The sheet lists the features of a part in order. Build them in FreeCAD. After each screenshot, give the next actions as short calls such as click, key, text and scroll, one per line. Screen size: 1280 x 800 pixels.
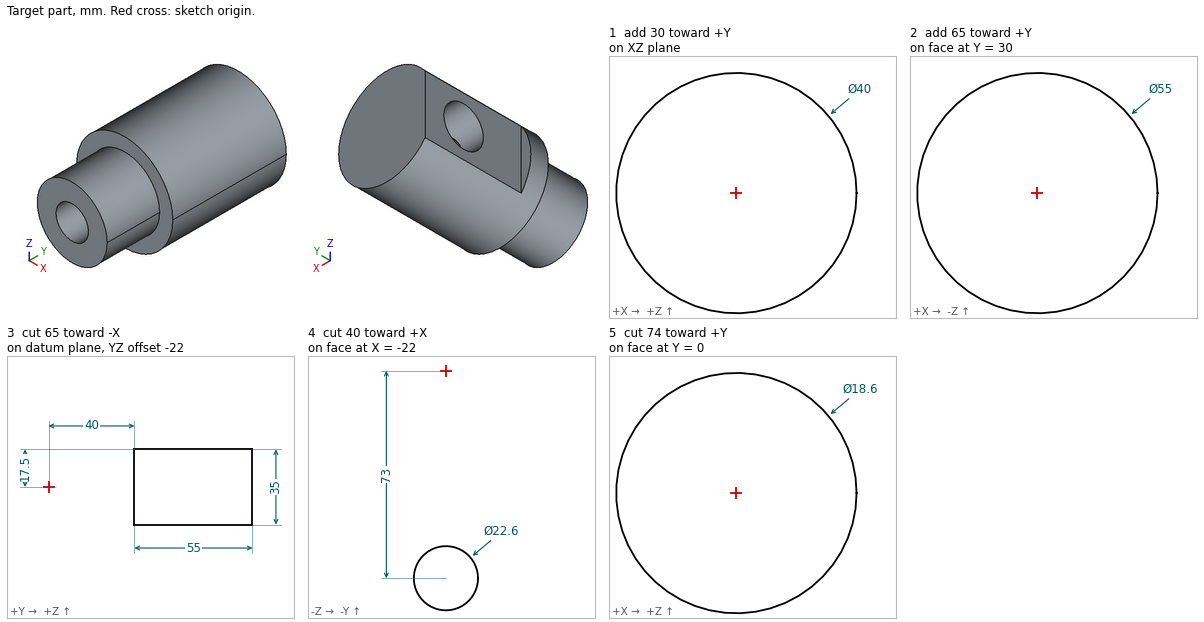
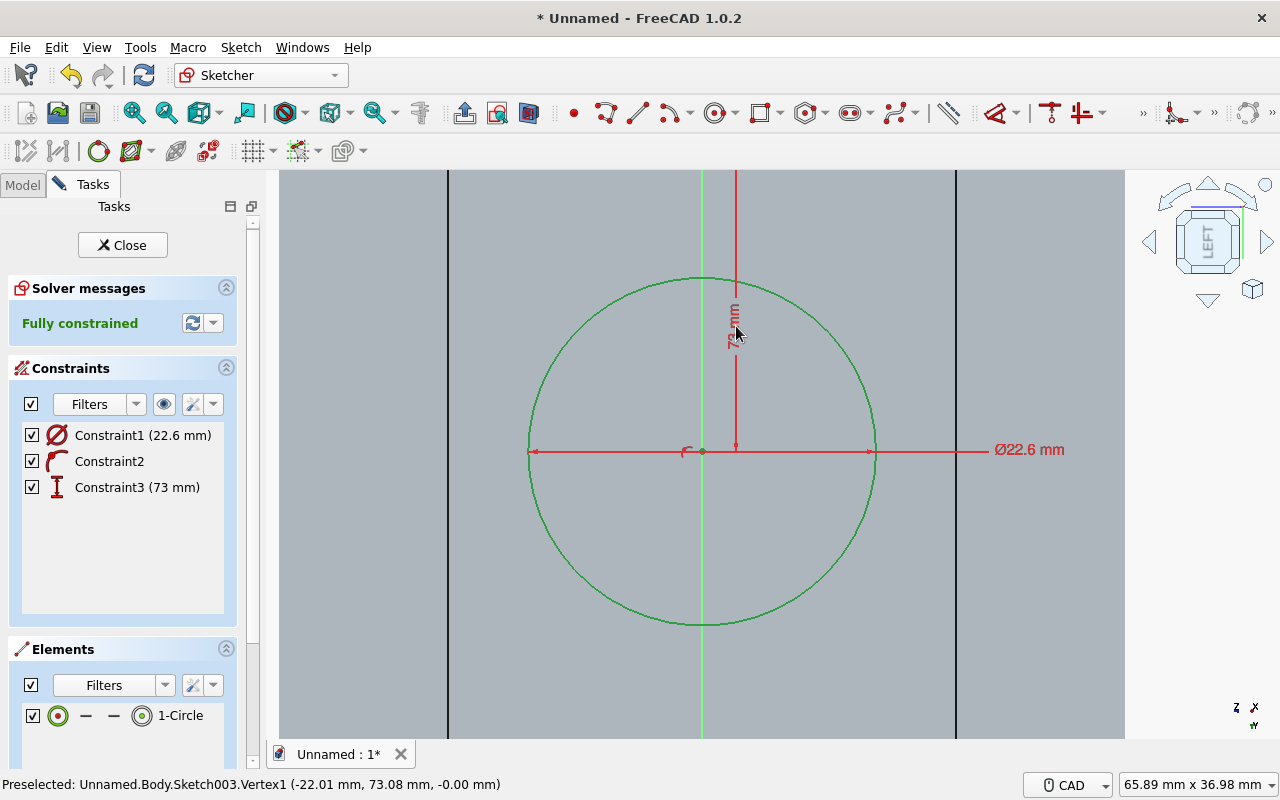
click(123, 245)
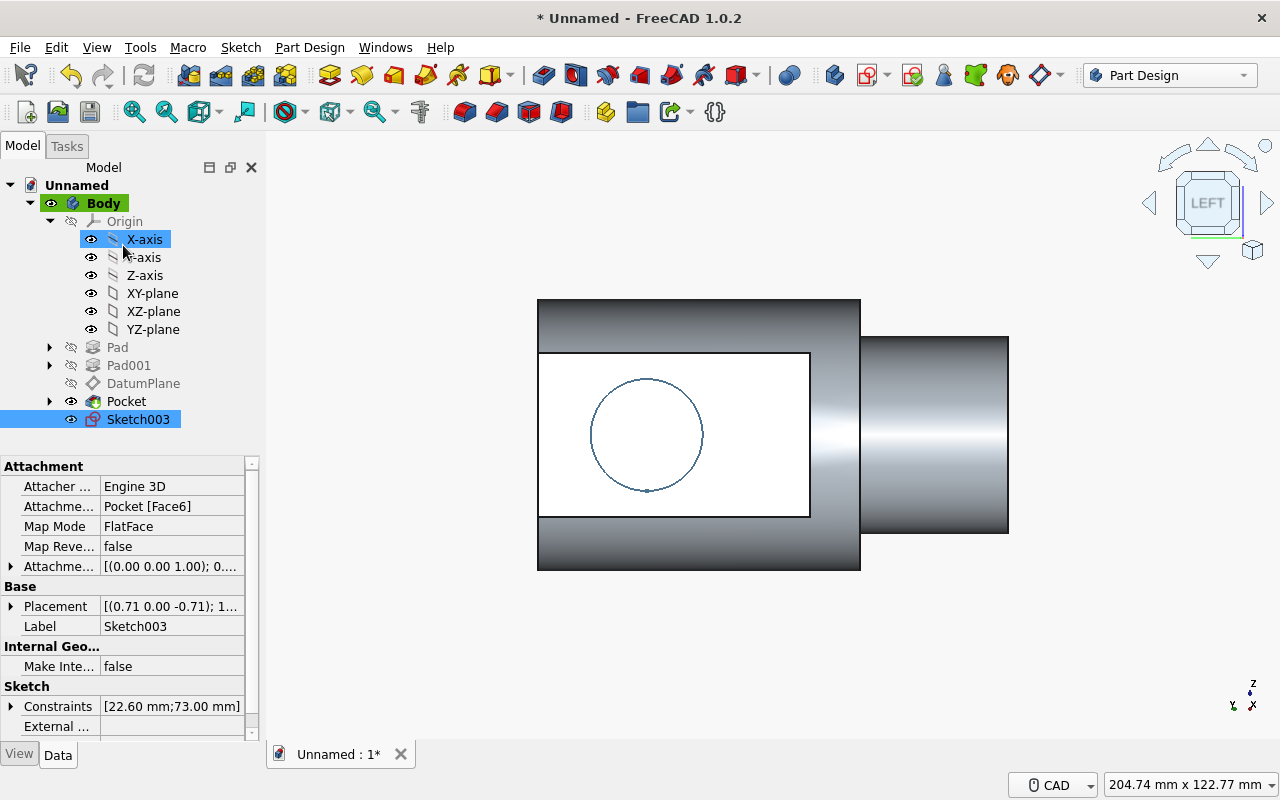
click(544, 76)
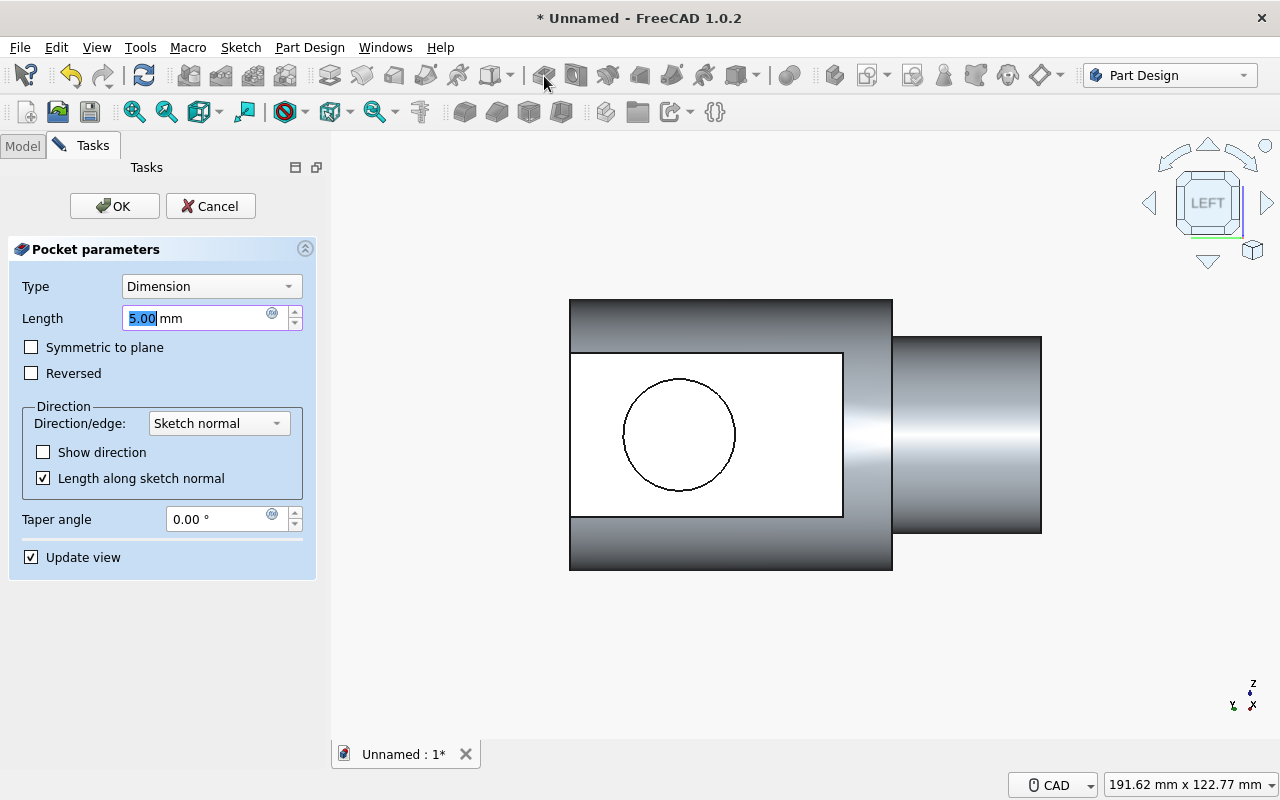
text(40)
key(Tab)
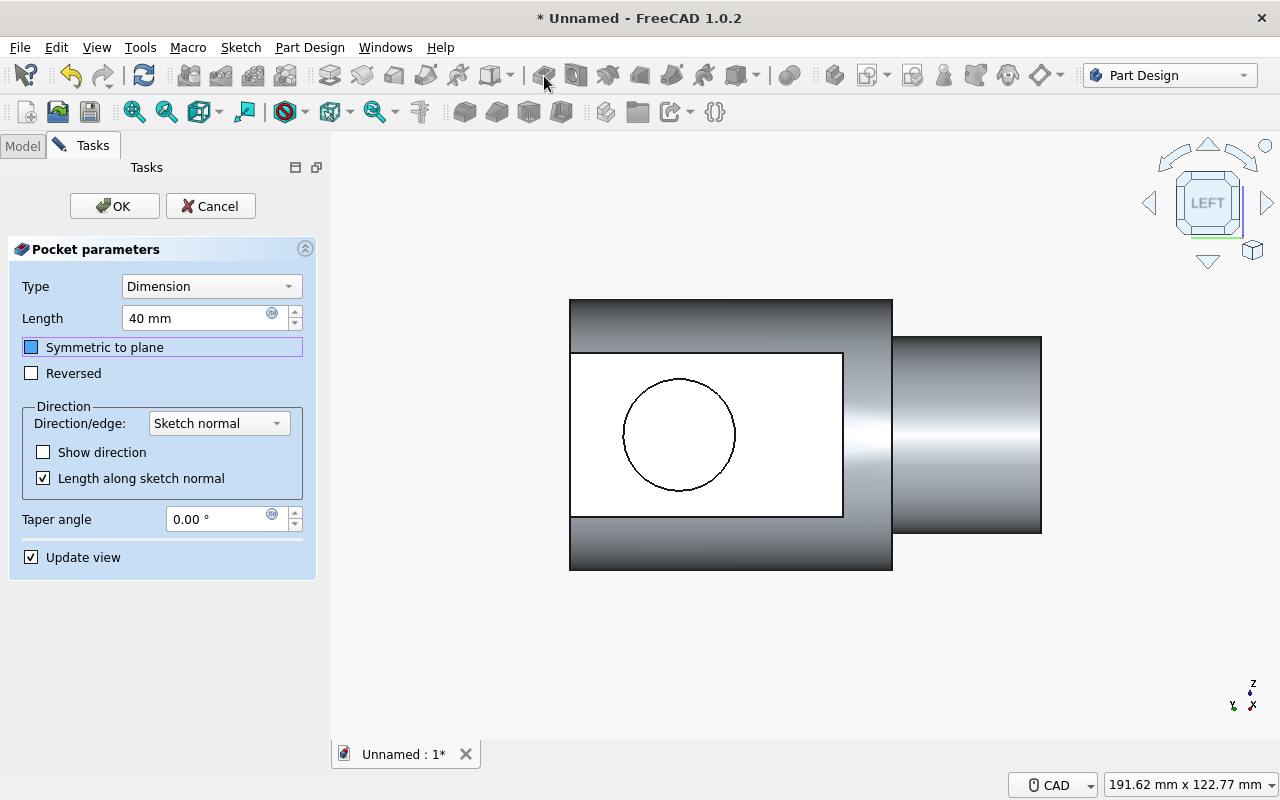
click(115, 206)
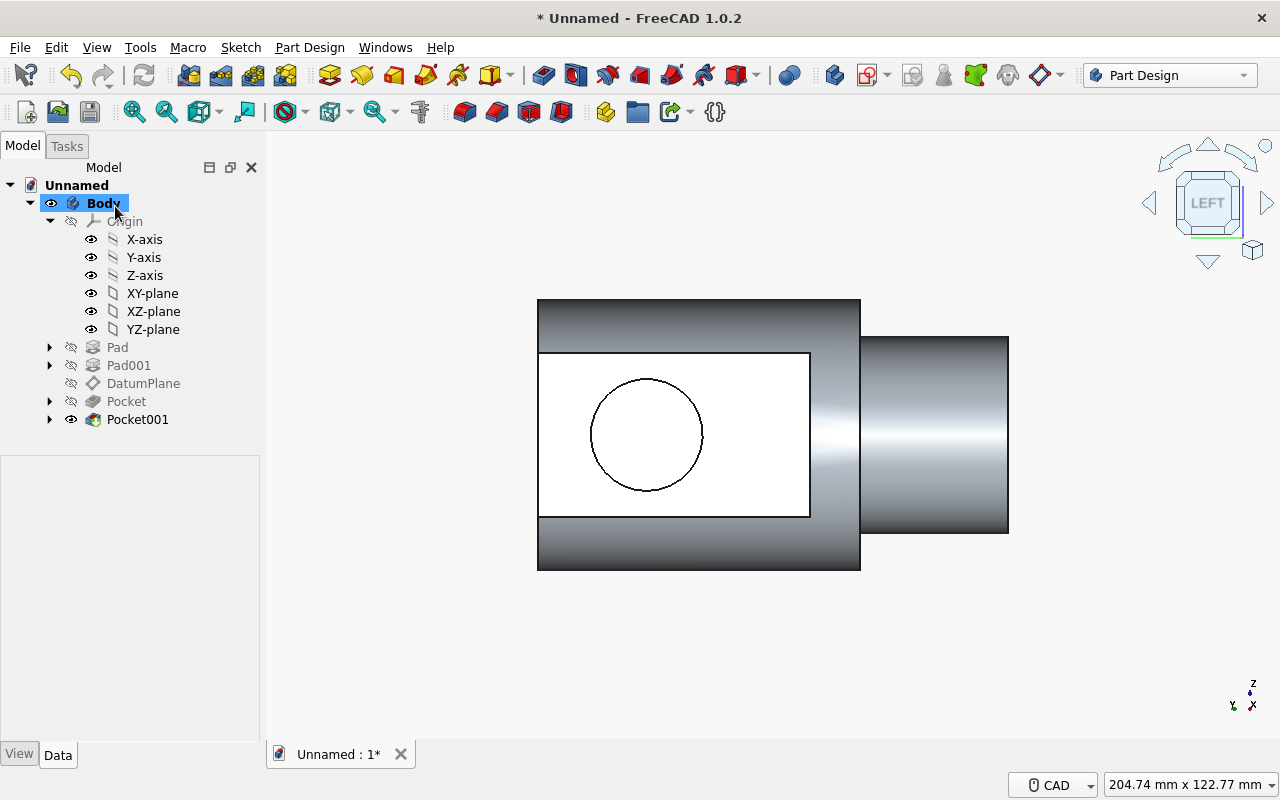
key(0)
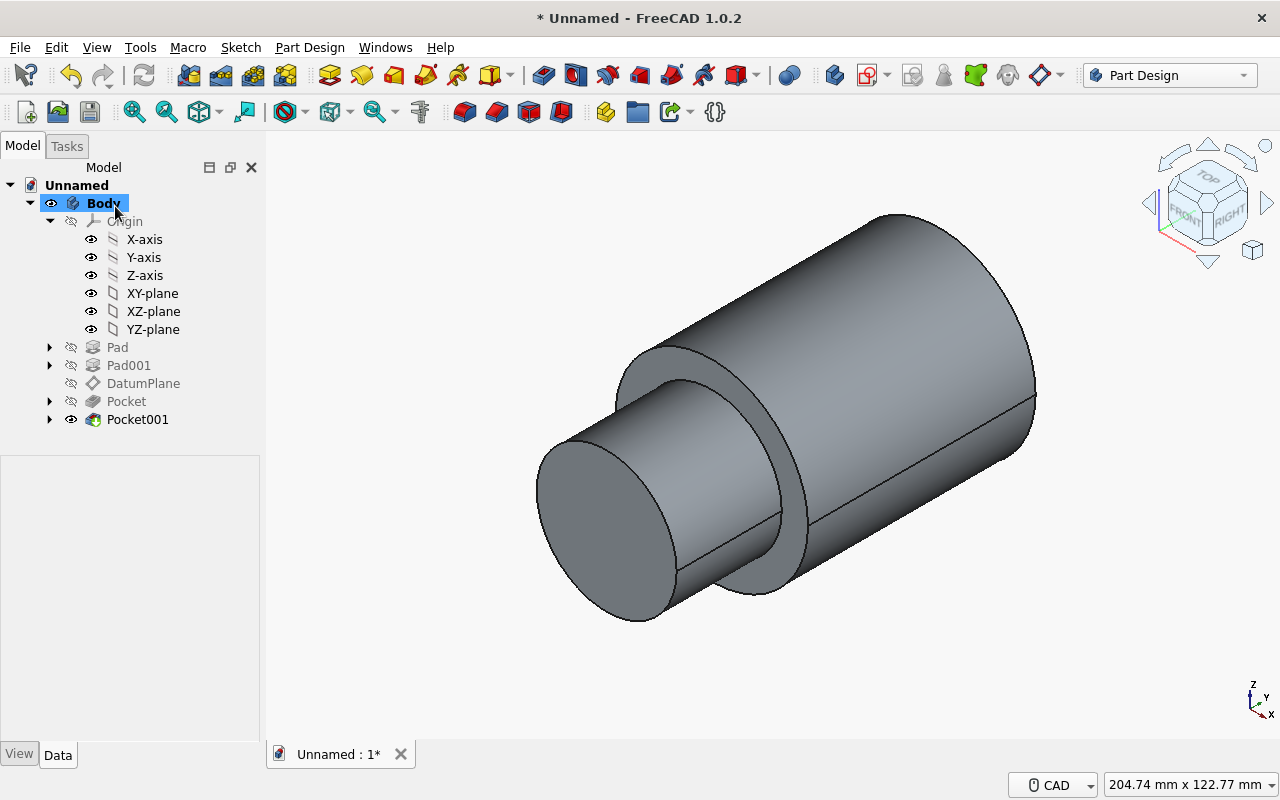
click(607, 530)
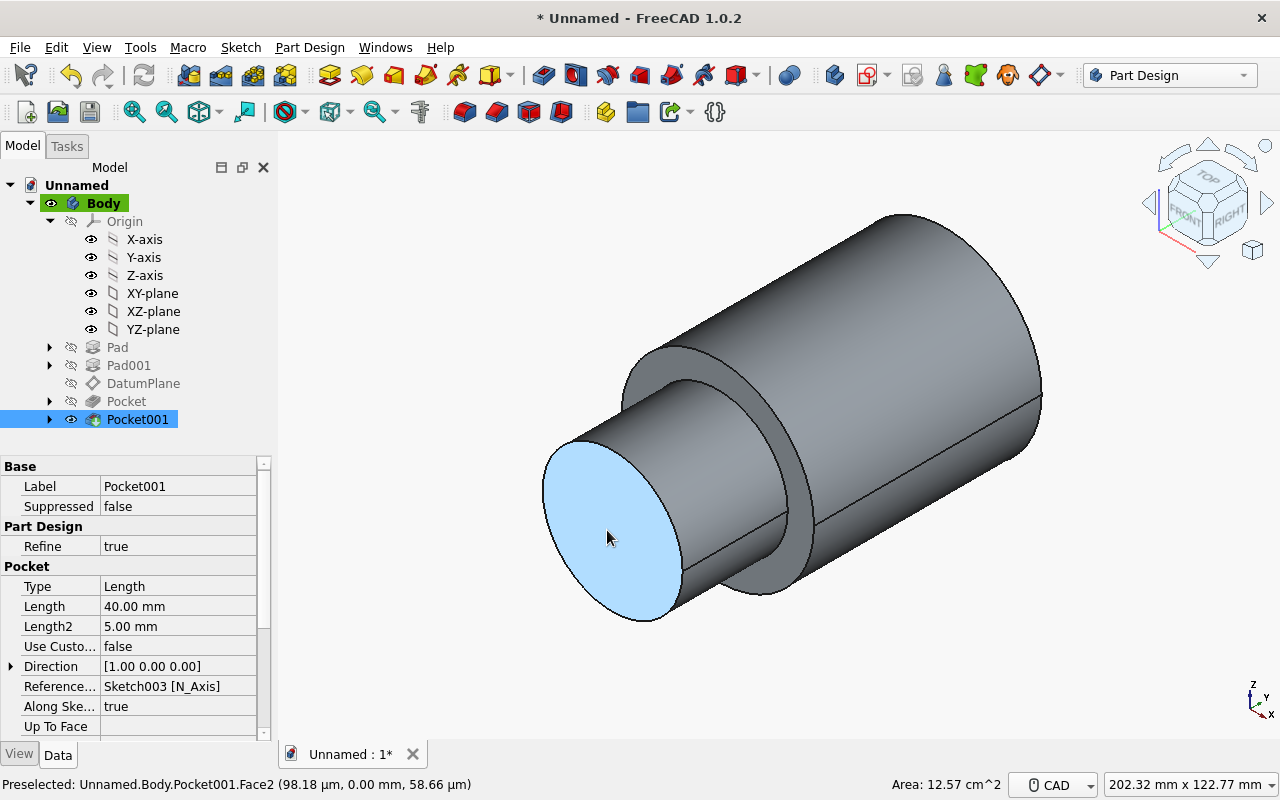
click(868, 76)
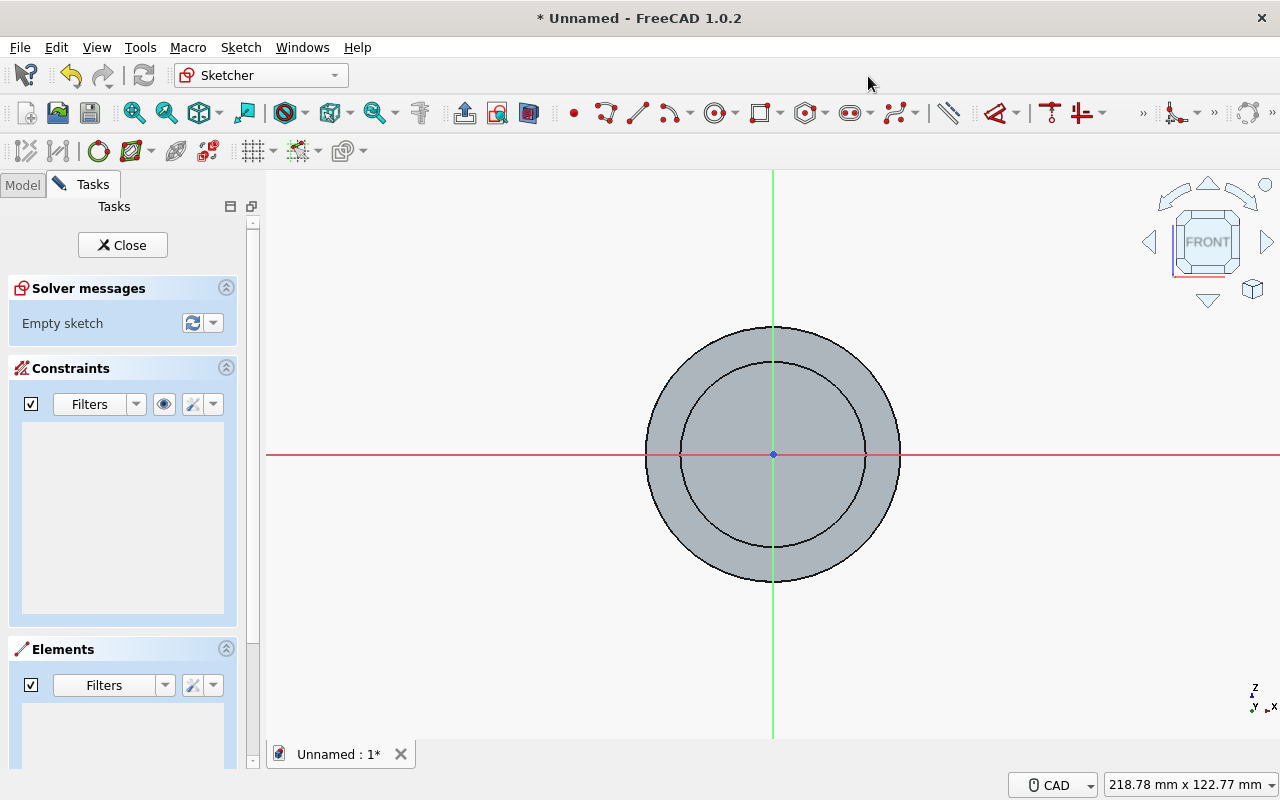
scroll(795, 455, up, 7)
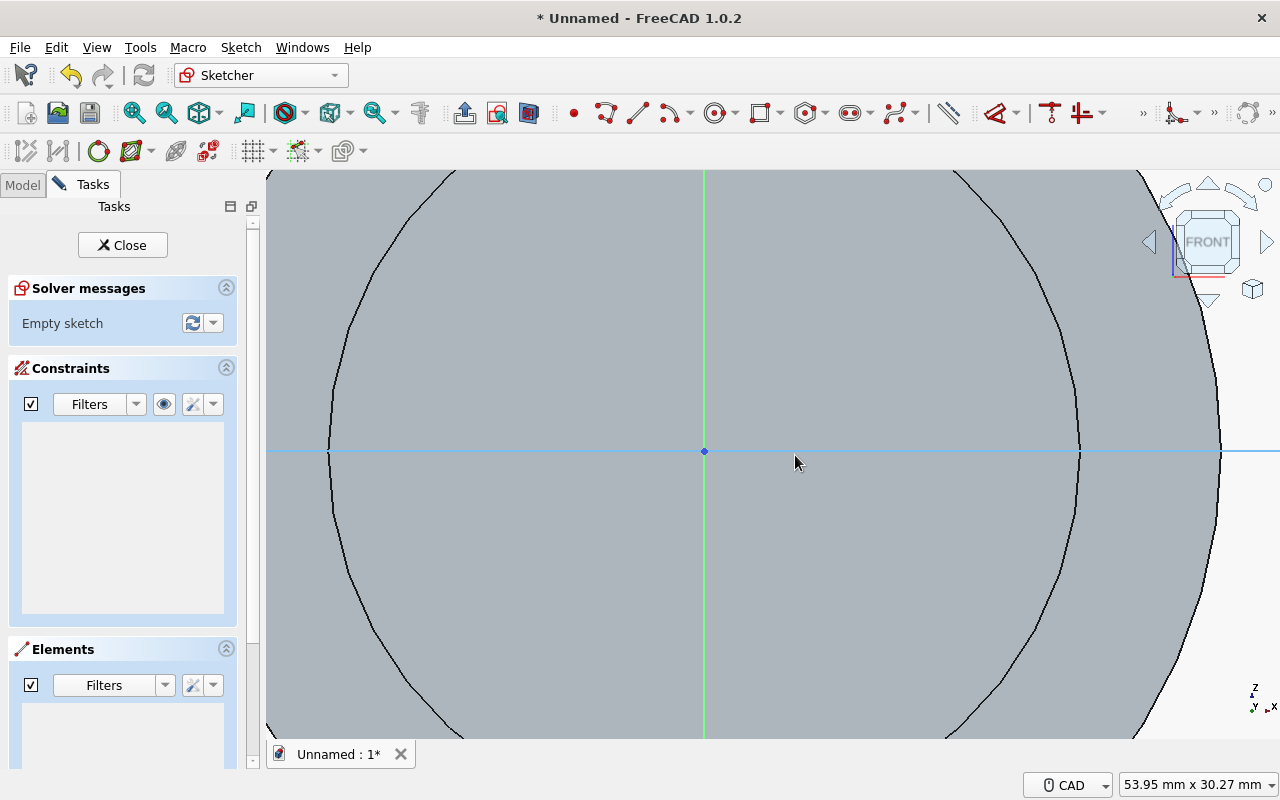
key(g)
key(c)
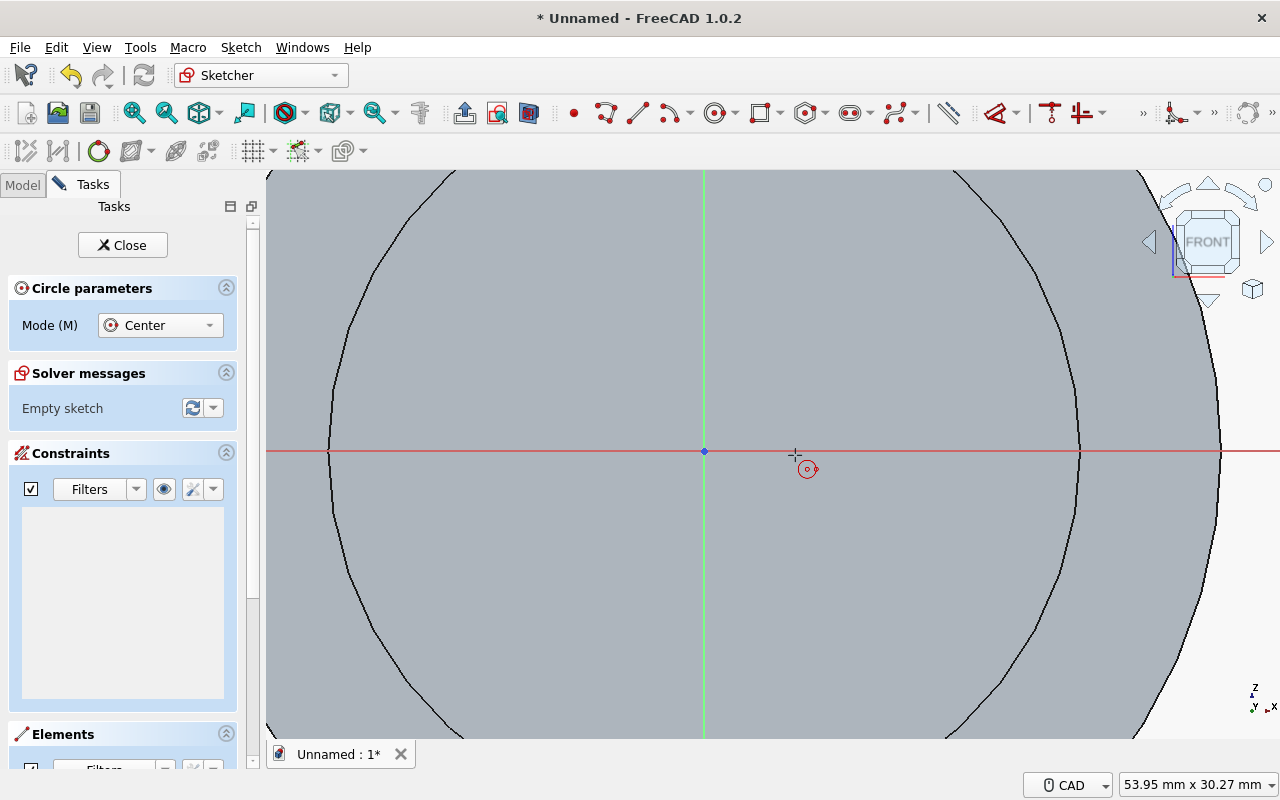
click(704, 451)
move(828, 328)